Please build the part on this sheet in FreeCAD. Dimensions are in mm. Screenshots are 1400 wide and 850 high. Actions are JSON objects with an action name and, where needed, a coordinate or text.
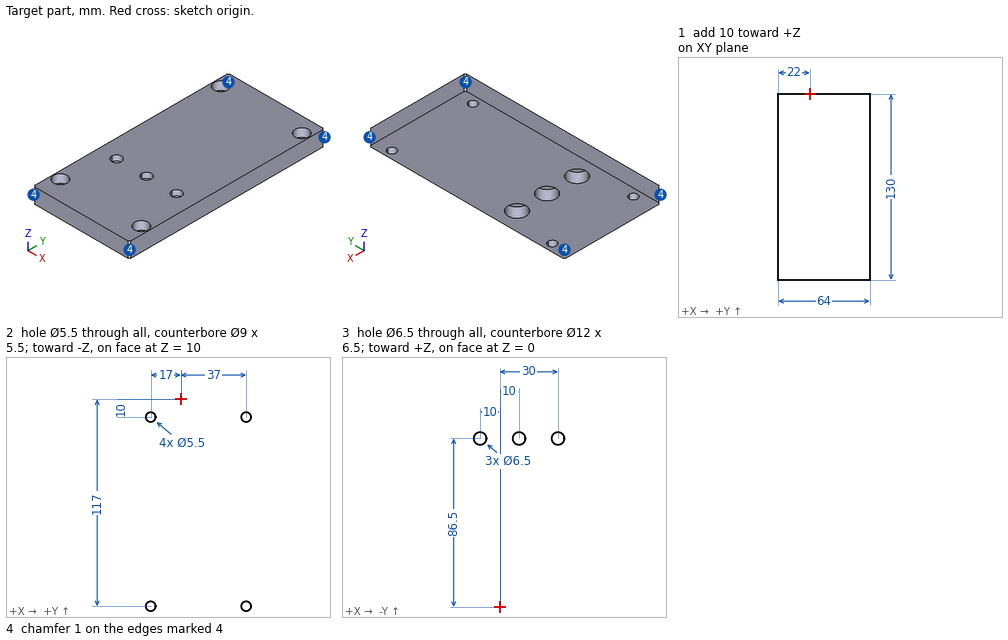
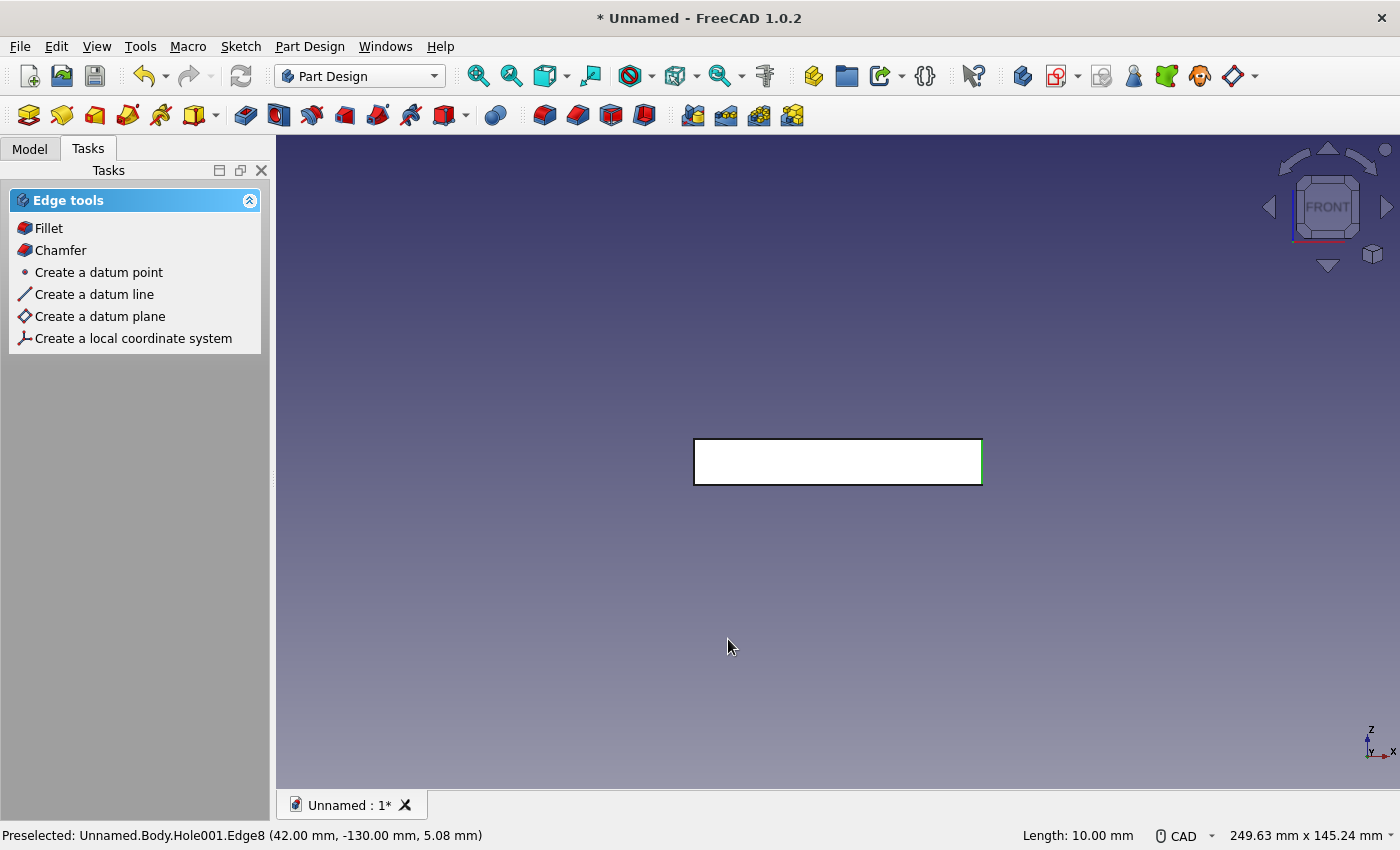
{"action": "left_click", "coordinate": [694, 461], "text": "ctrl"}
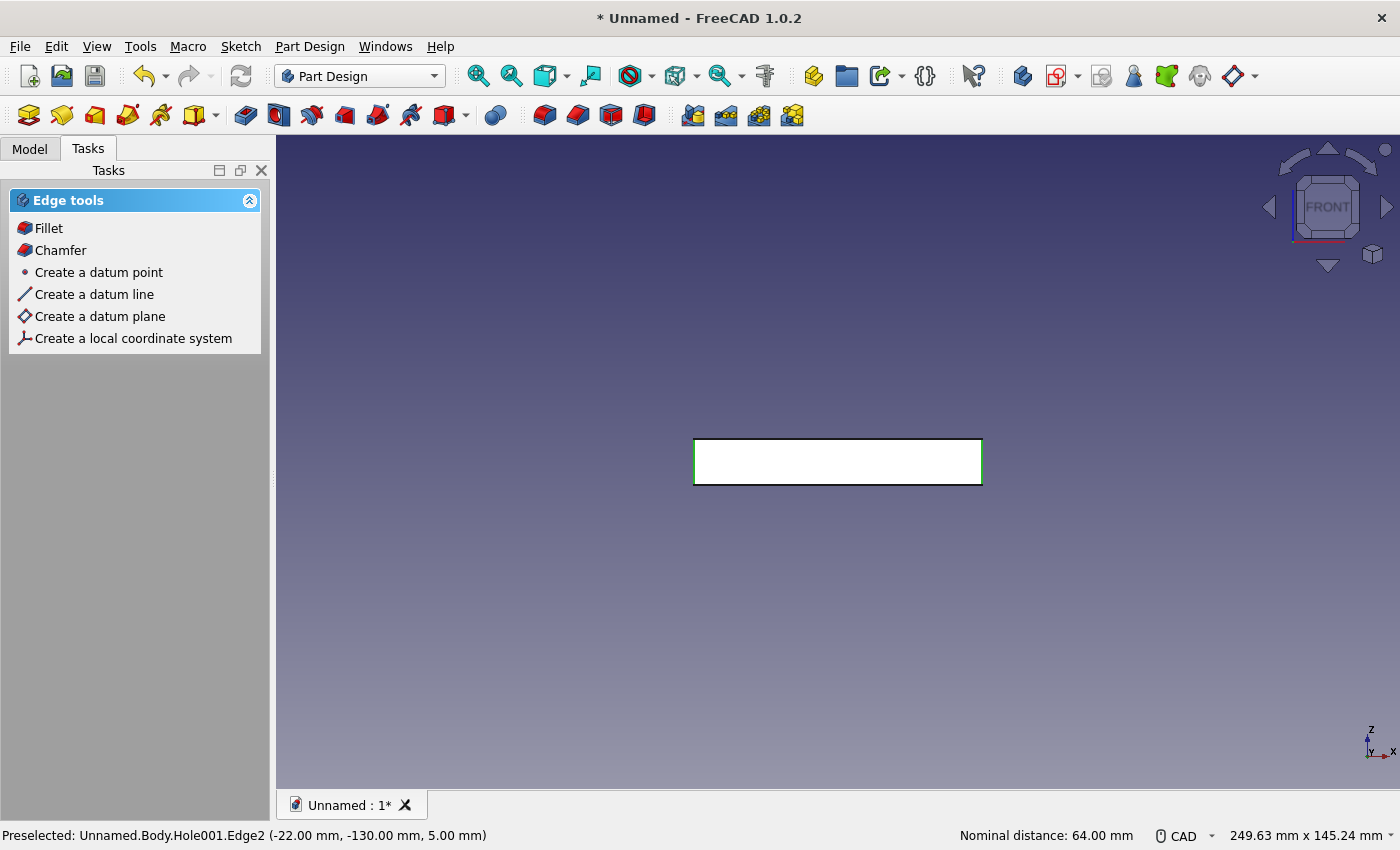
{"action": "key", "text": "3"}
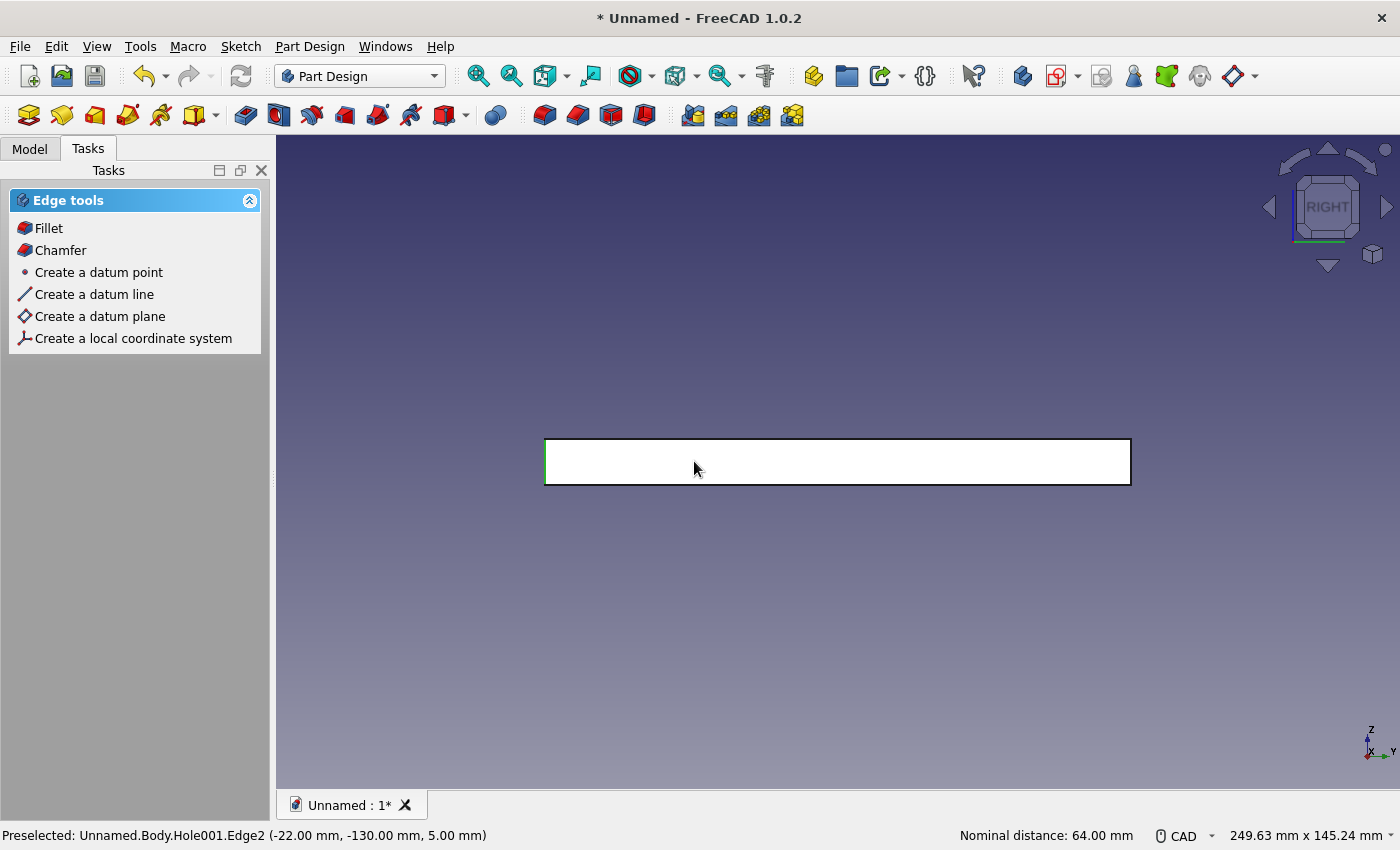
{"action": "left_click", "coordinate": [1131, 461], "text": "ctrl"}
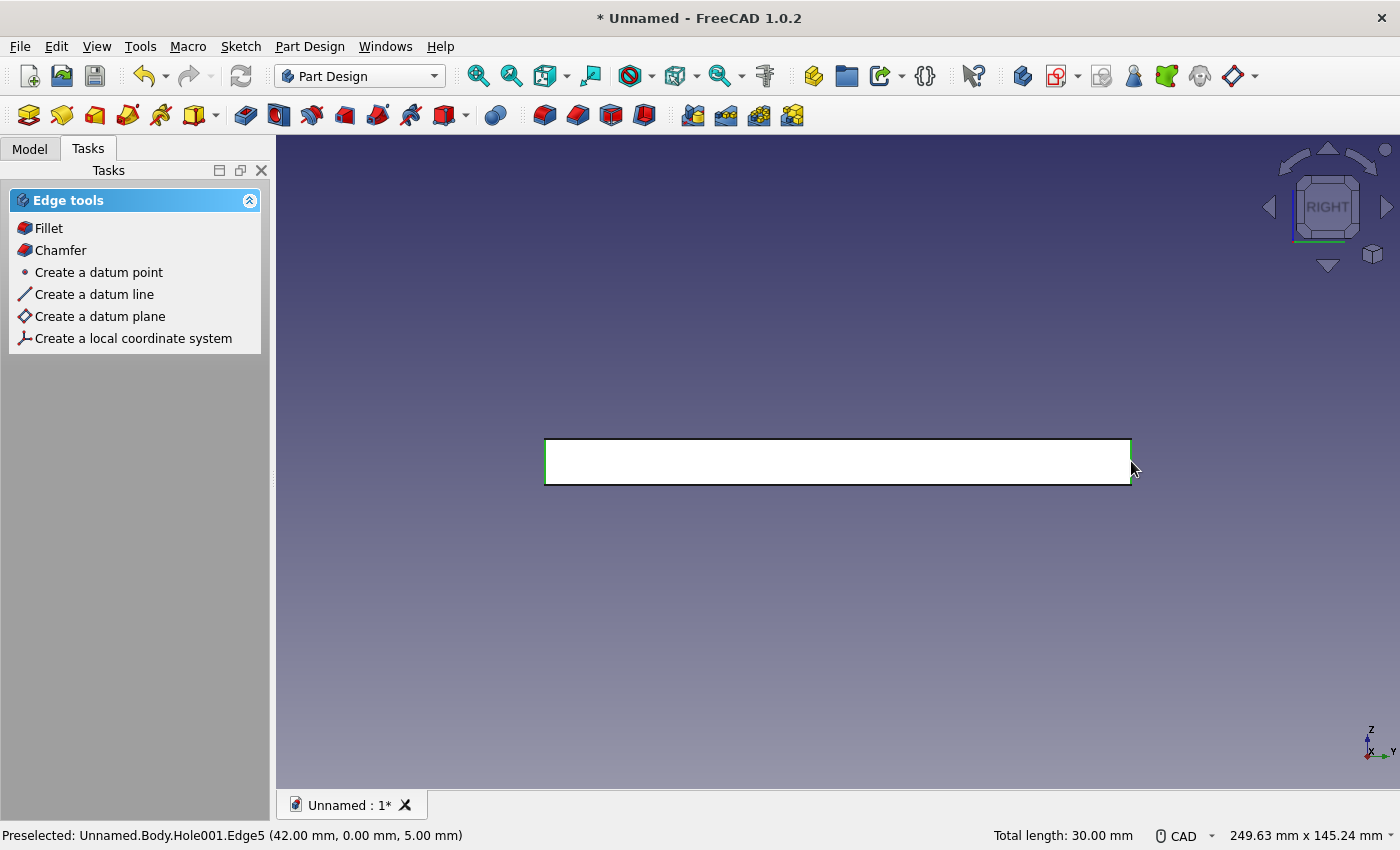
{"action": "key", "text": "5"}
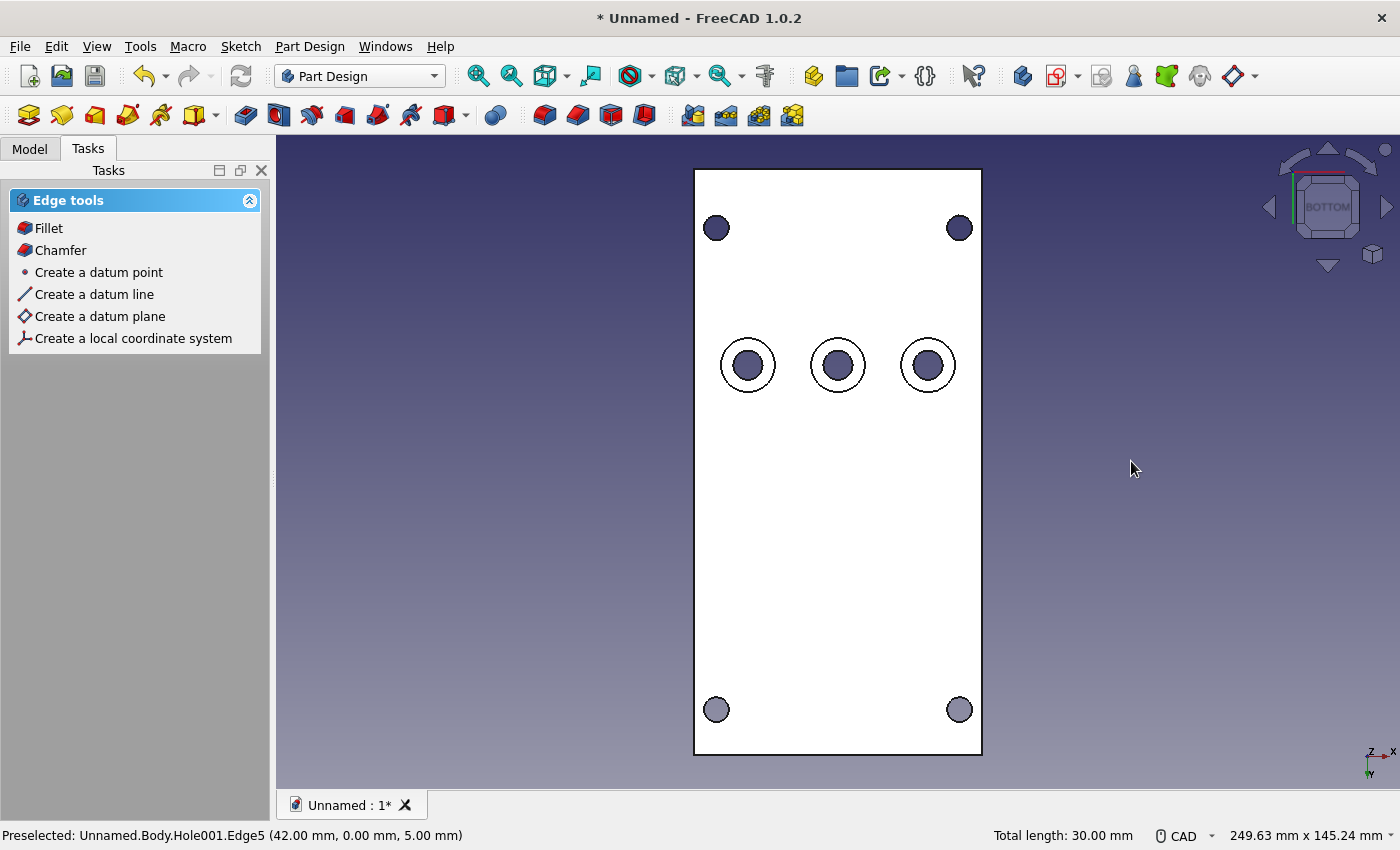
{"action": "key", "text": "4"}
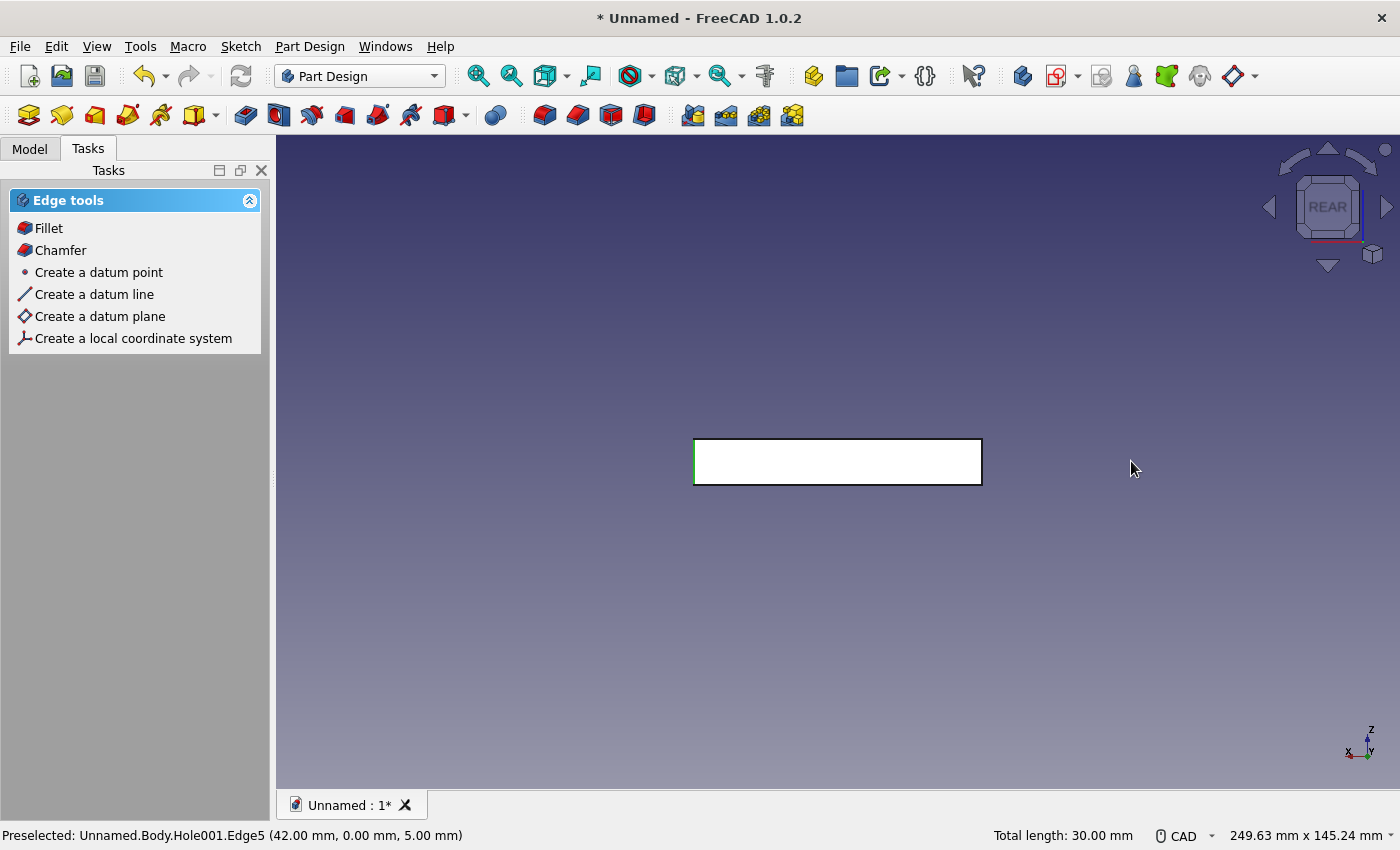
{"action": "key", "text": "v f"}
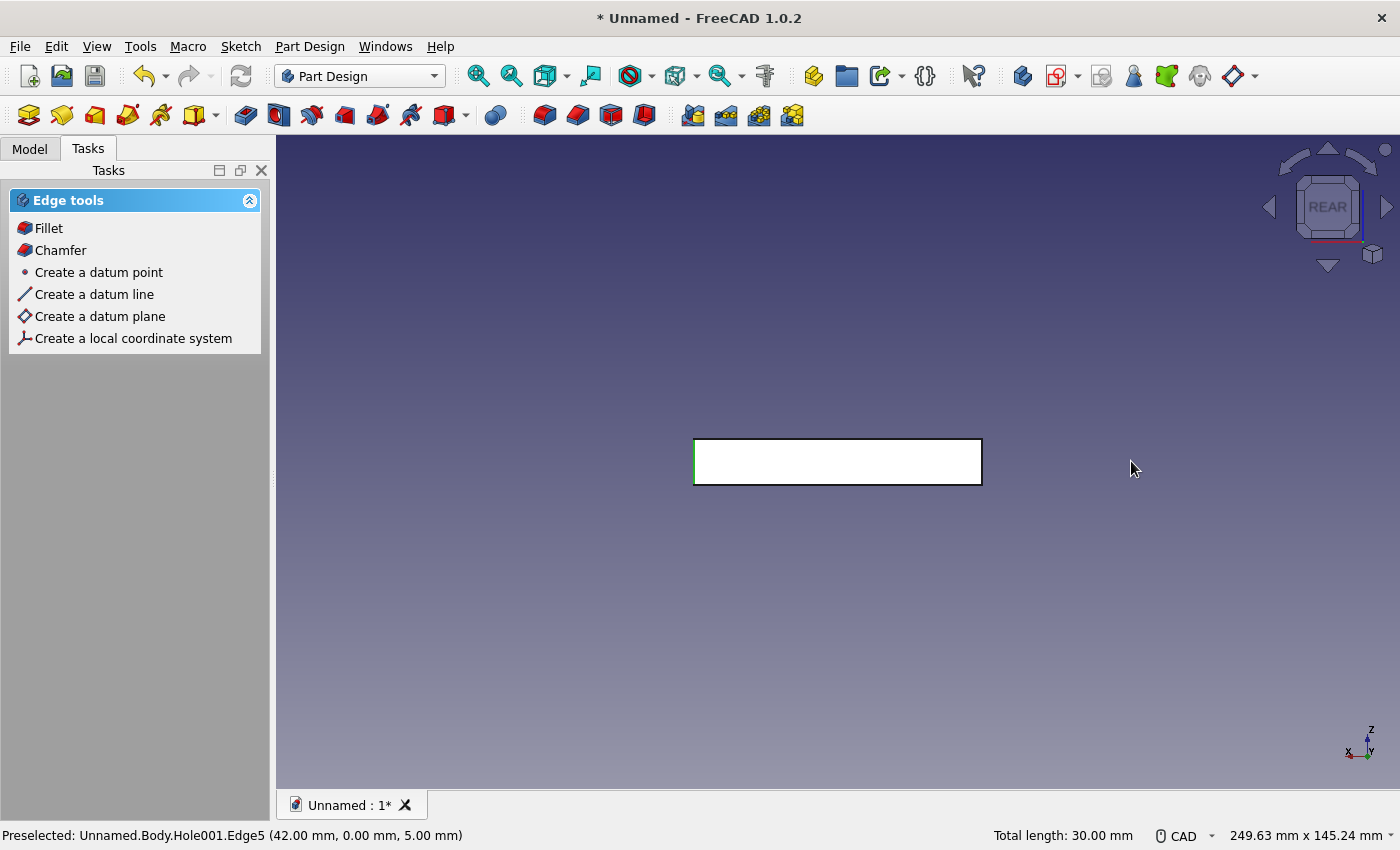
{"action": "left_click", "coordinate": [982, 461], "text": "ctrl"}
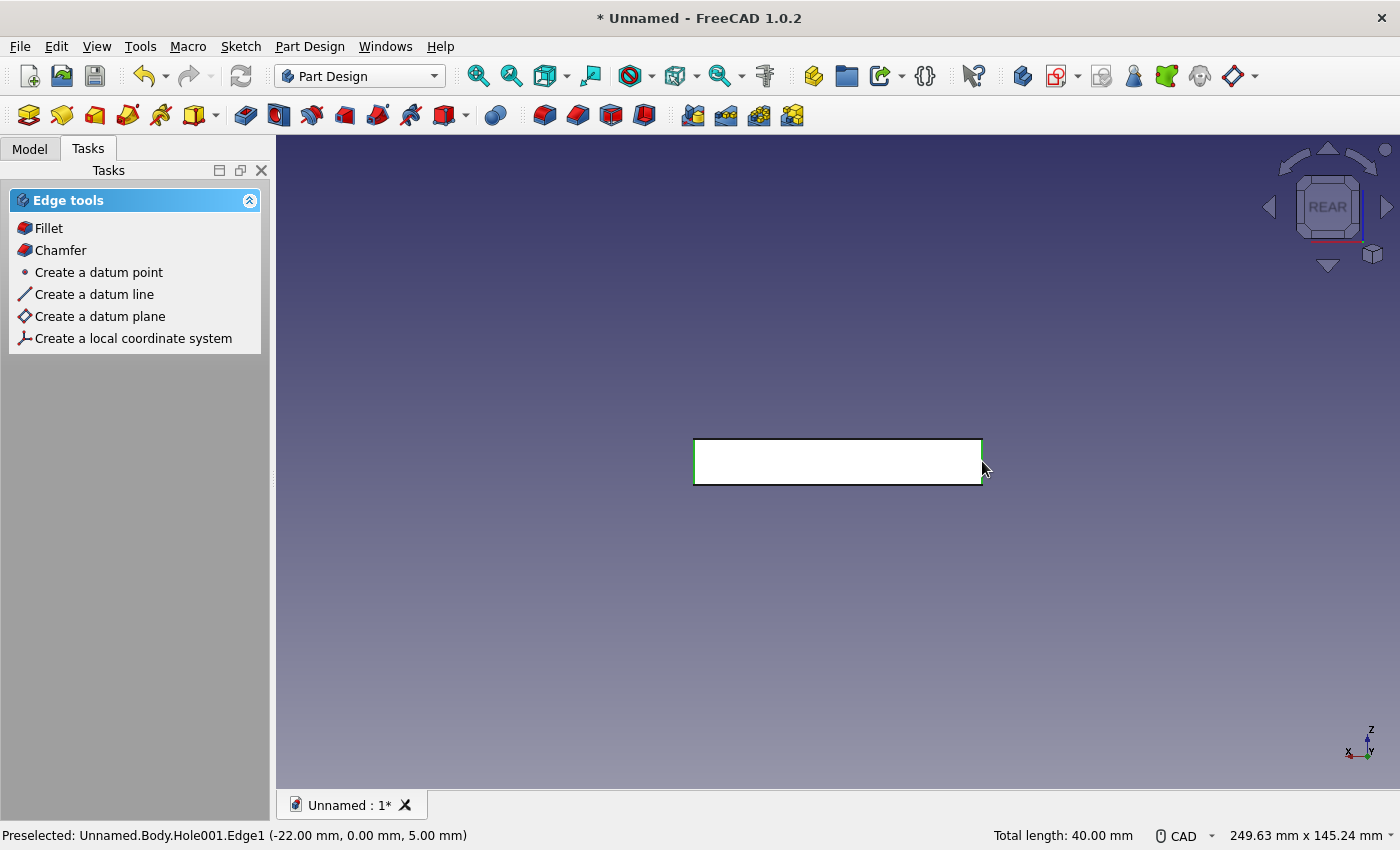
{"action": "left_click", "coordinate": [578, 116]}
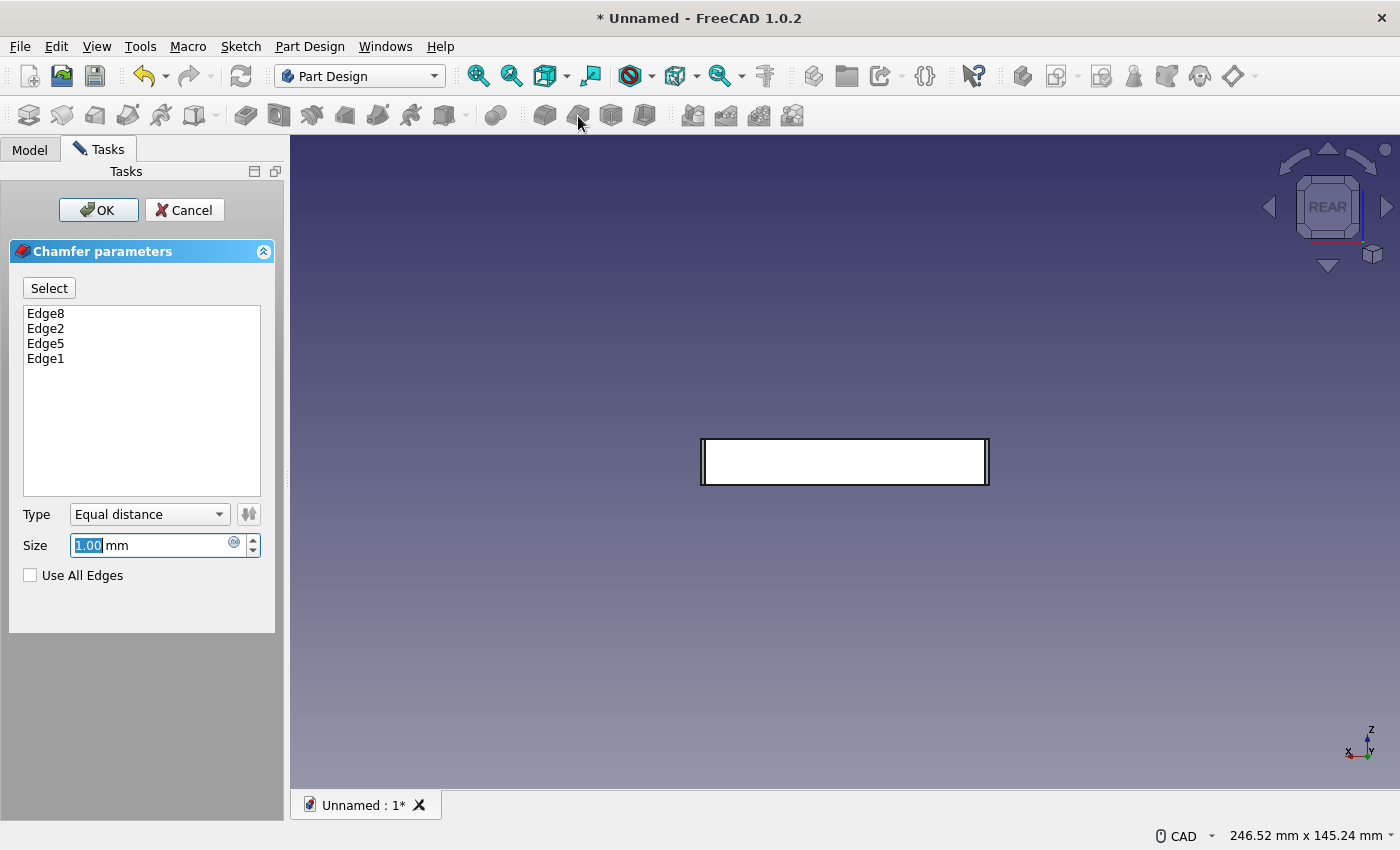
{"action": "type", "text": "1"}
{"action": "key", "text": "Tab"}